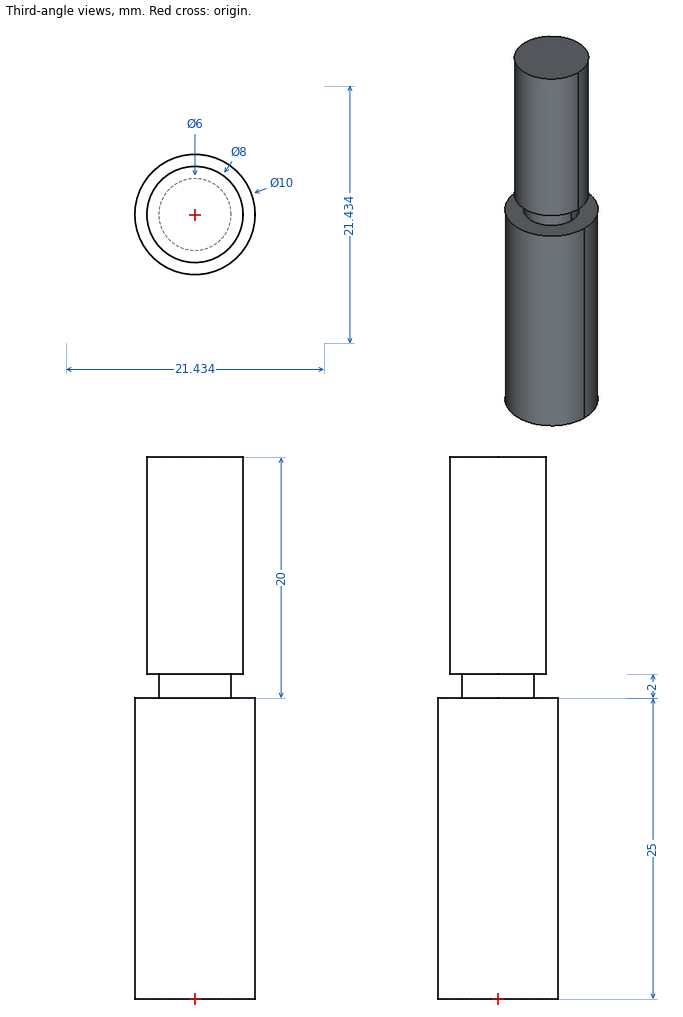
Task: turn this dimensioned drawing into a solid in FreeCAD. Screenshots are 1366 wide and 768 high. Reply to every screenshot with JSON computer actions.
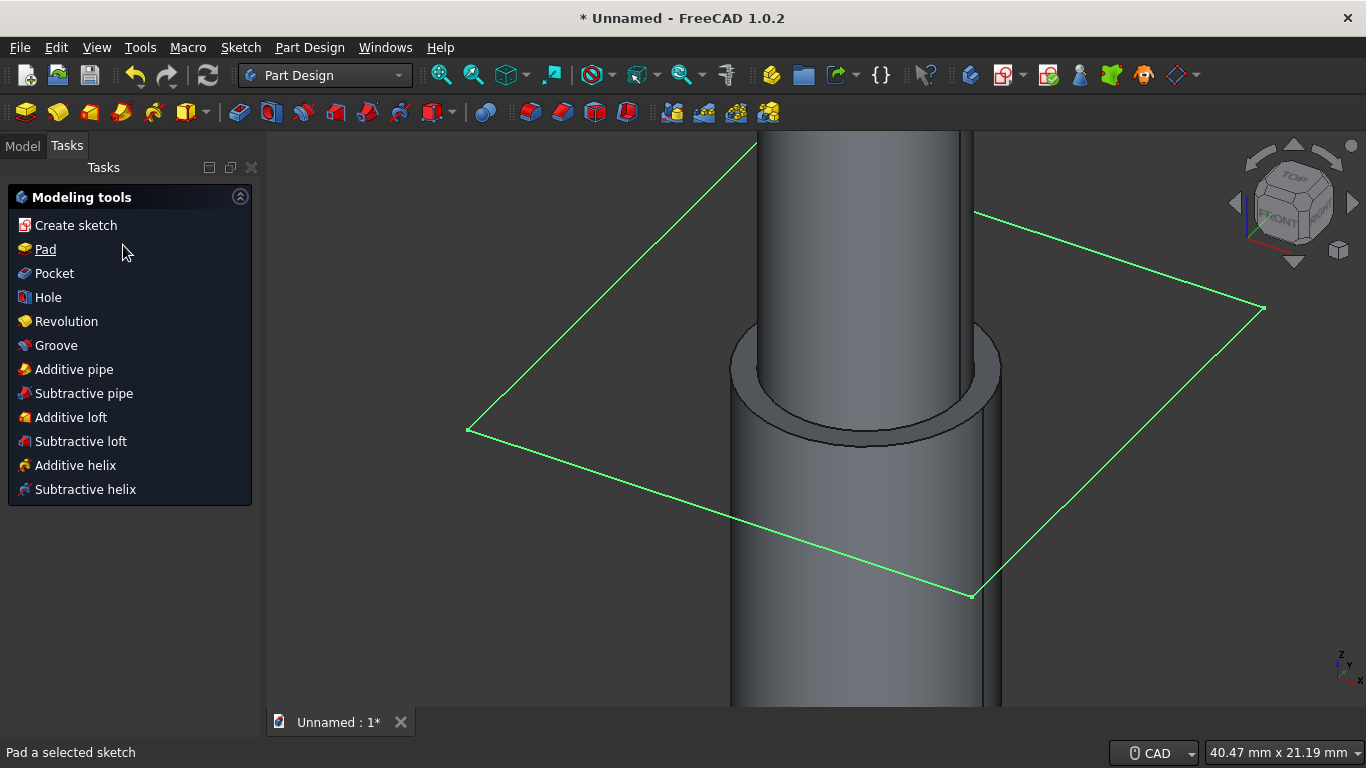
{"action": "left_click", "coordinate": [240, 112]}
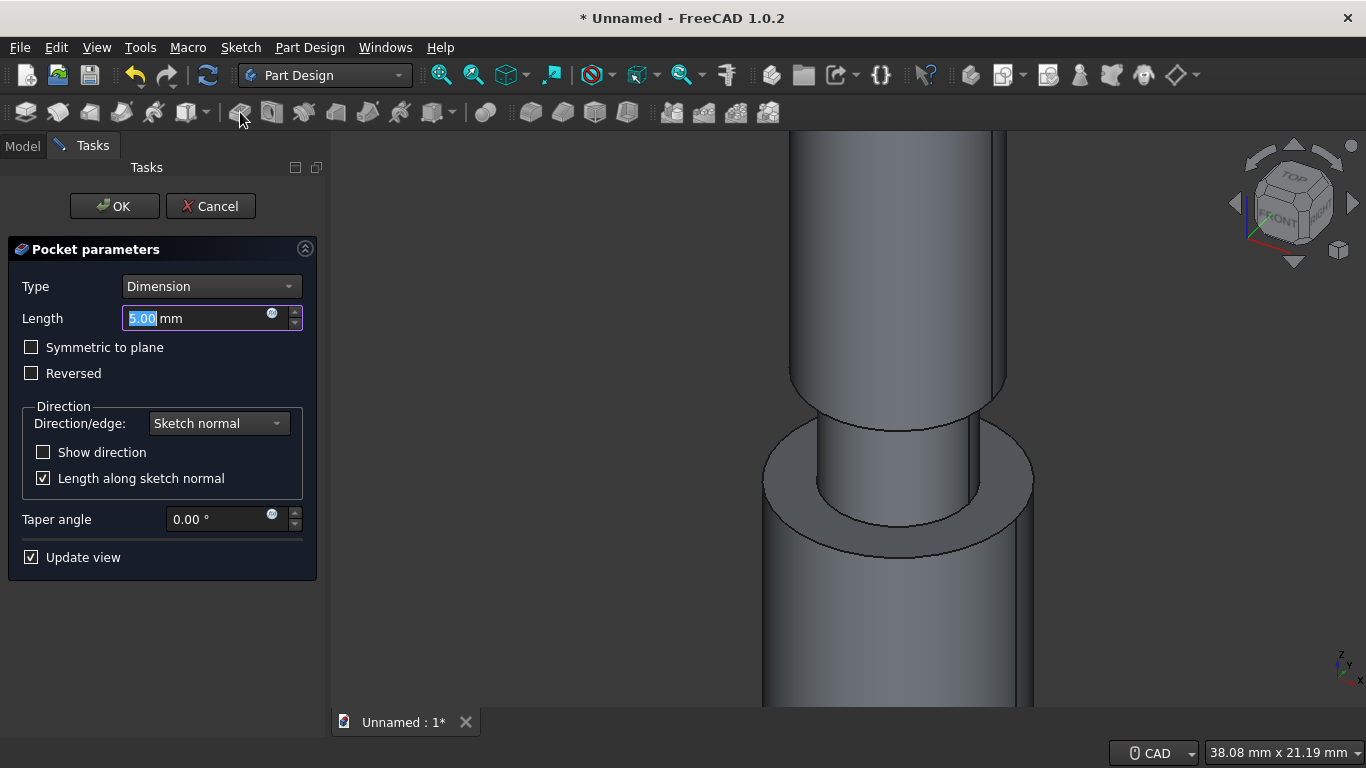
{"action": "type", "text": "2"}
{"action": "key", "text": "Tab"}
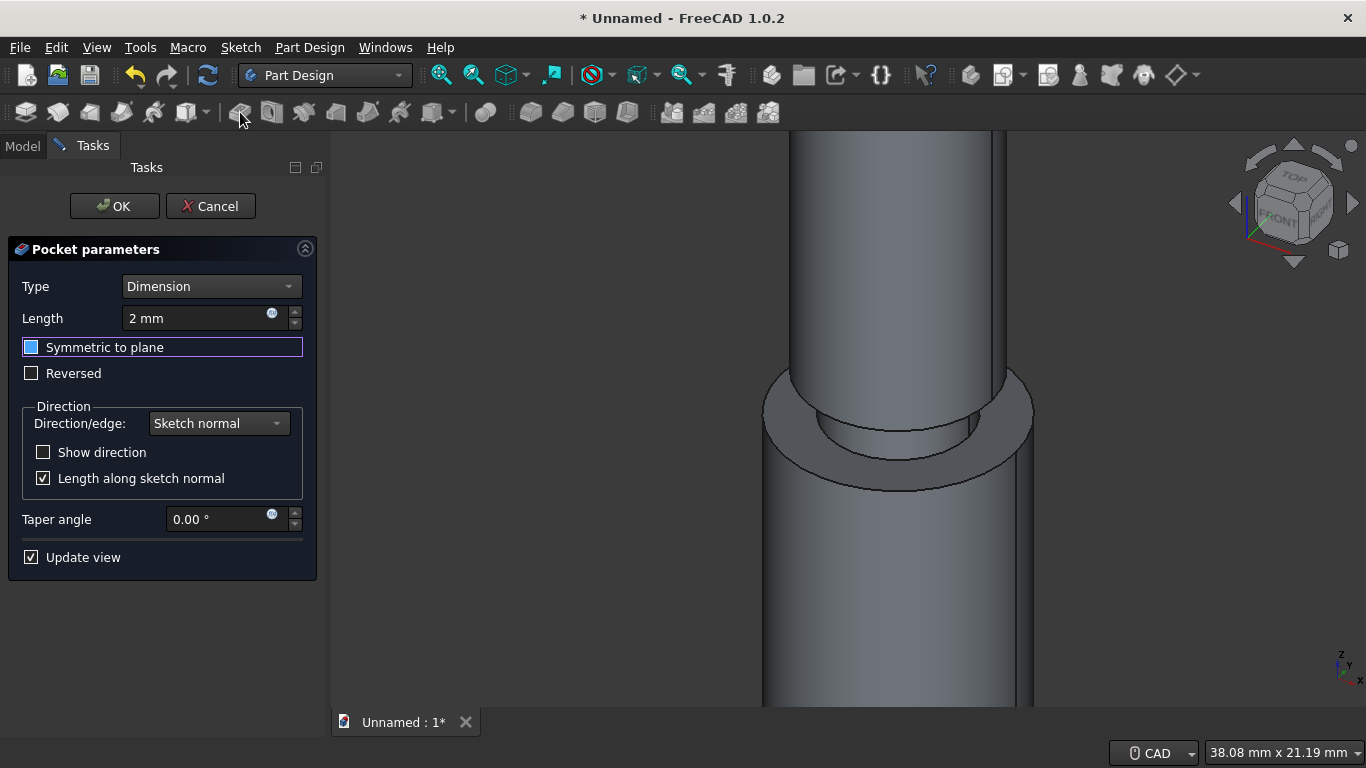
{"action": "left_click", "coordinate": [30, 373]}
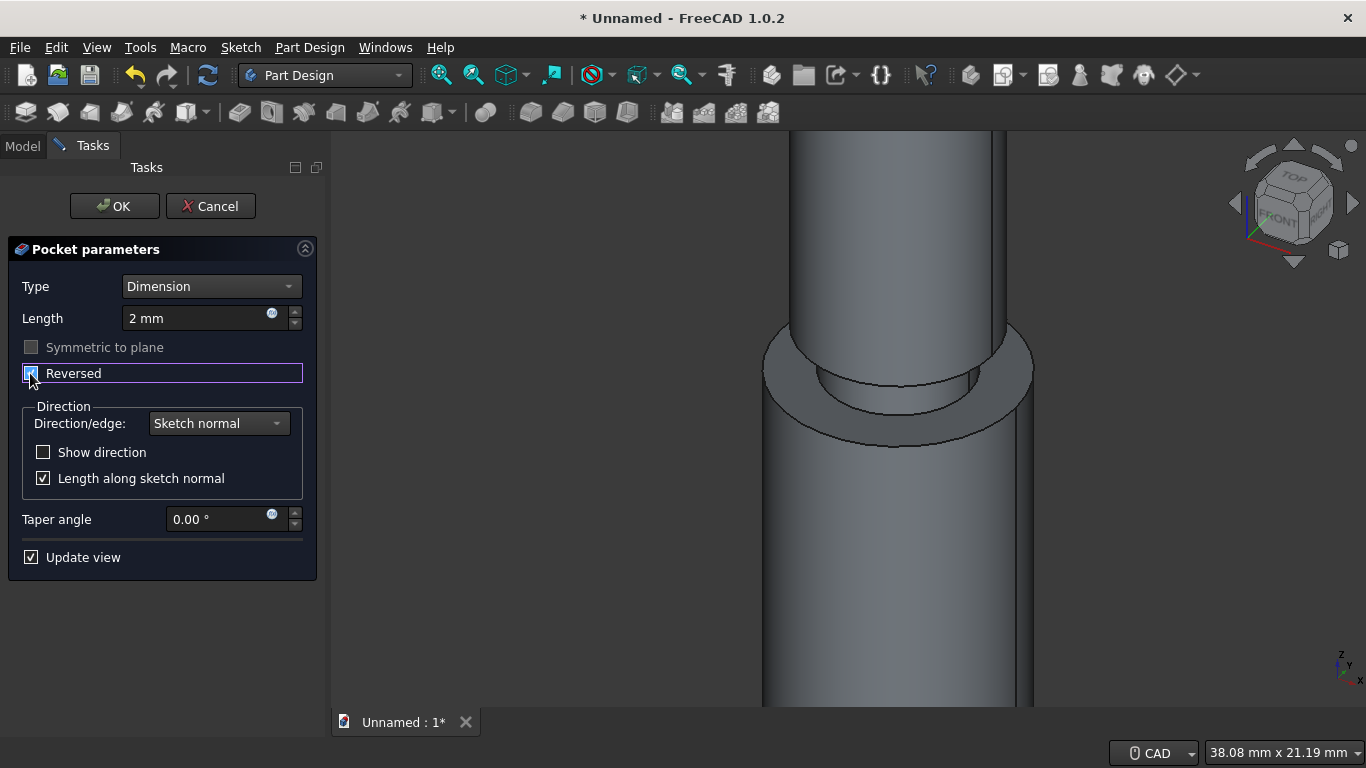
{"action": "left_click", "coordinate": [115, 206]}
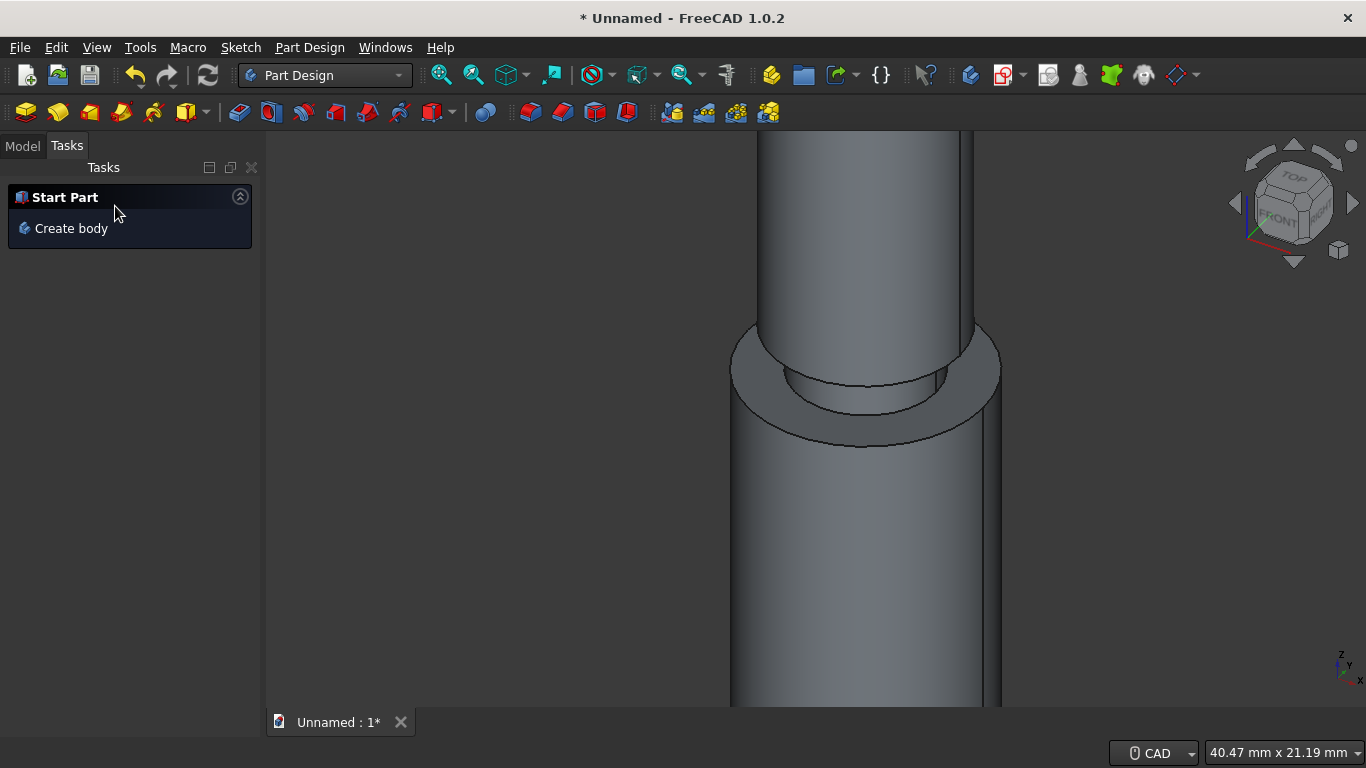
{"action": "key", "text": "0"}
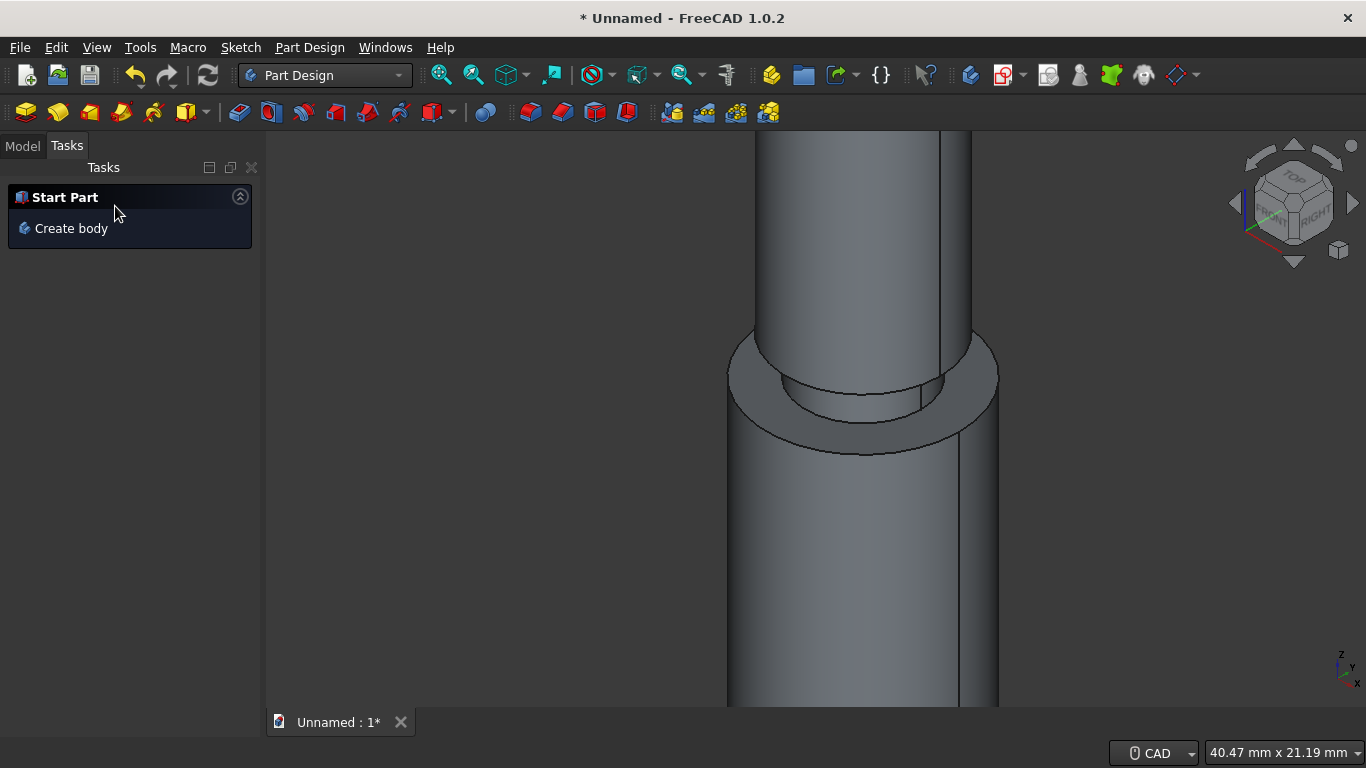
{"action": "left_click", "coordinate": [442, 76]}